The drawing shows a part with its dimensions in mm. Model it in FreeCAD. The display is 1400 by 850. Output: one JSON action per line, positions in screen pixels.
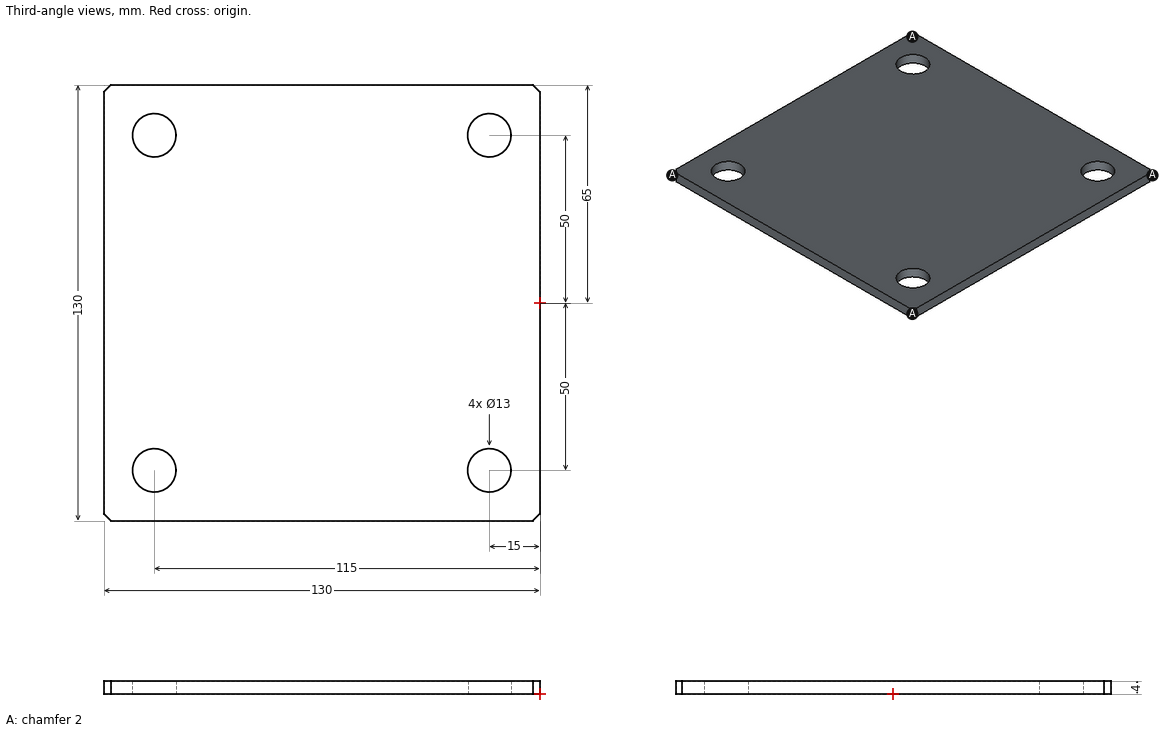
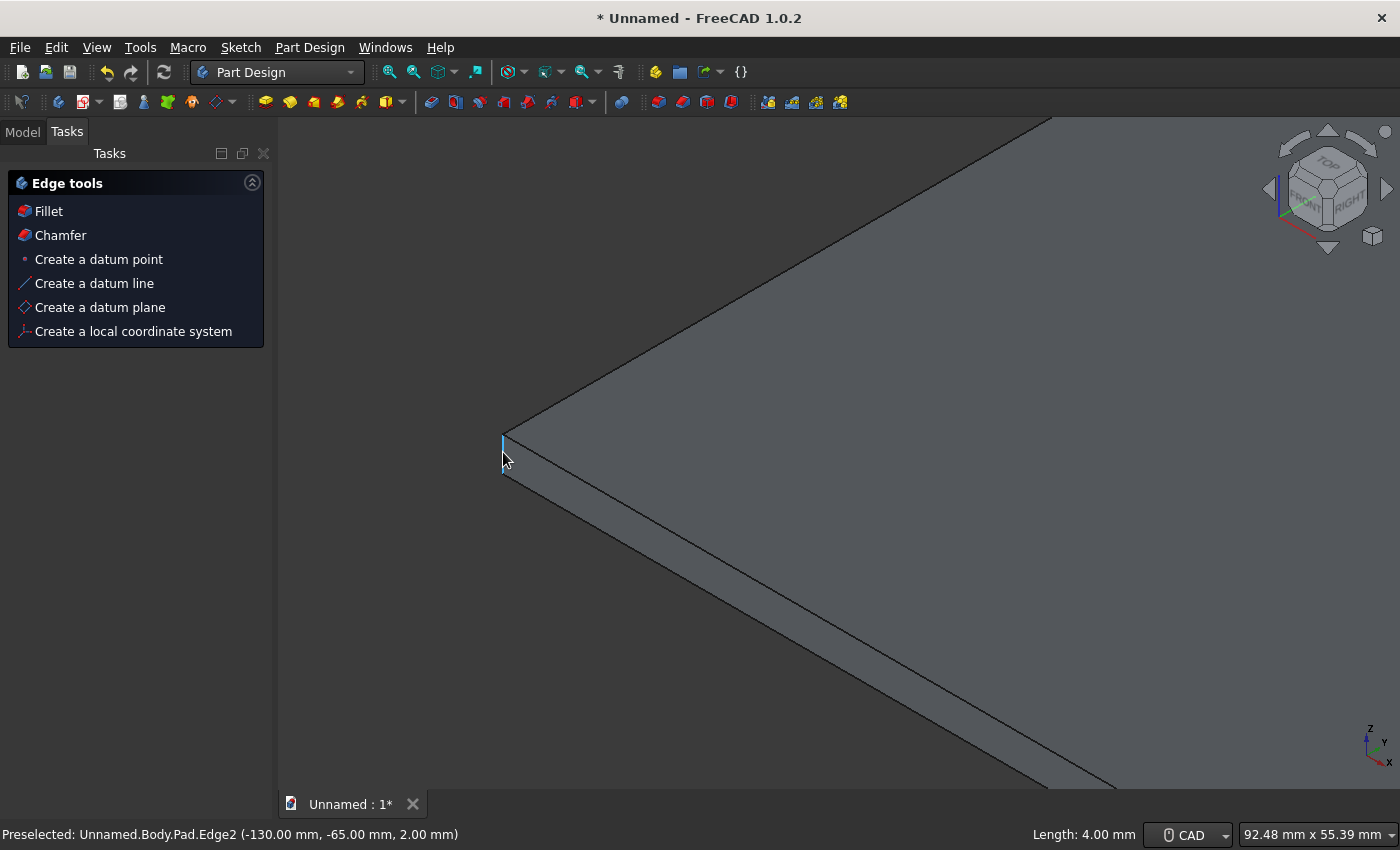
{"action": "left_click", "coordinate": [390, 72]}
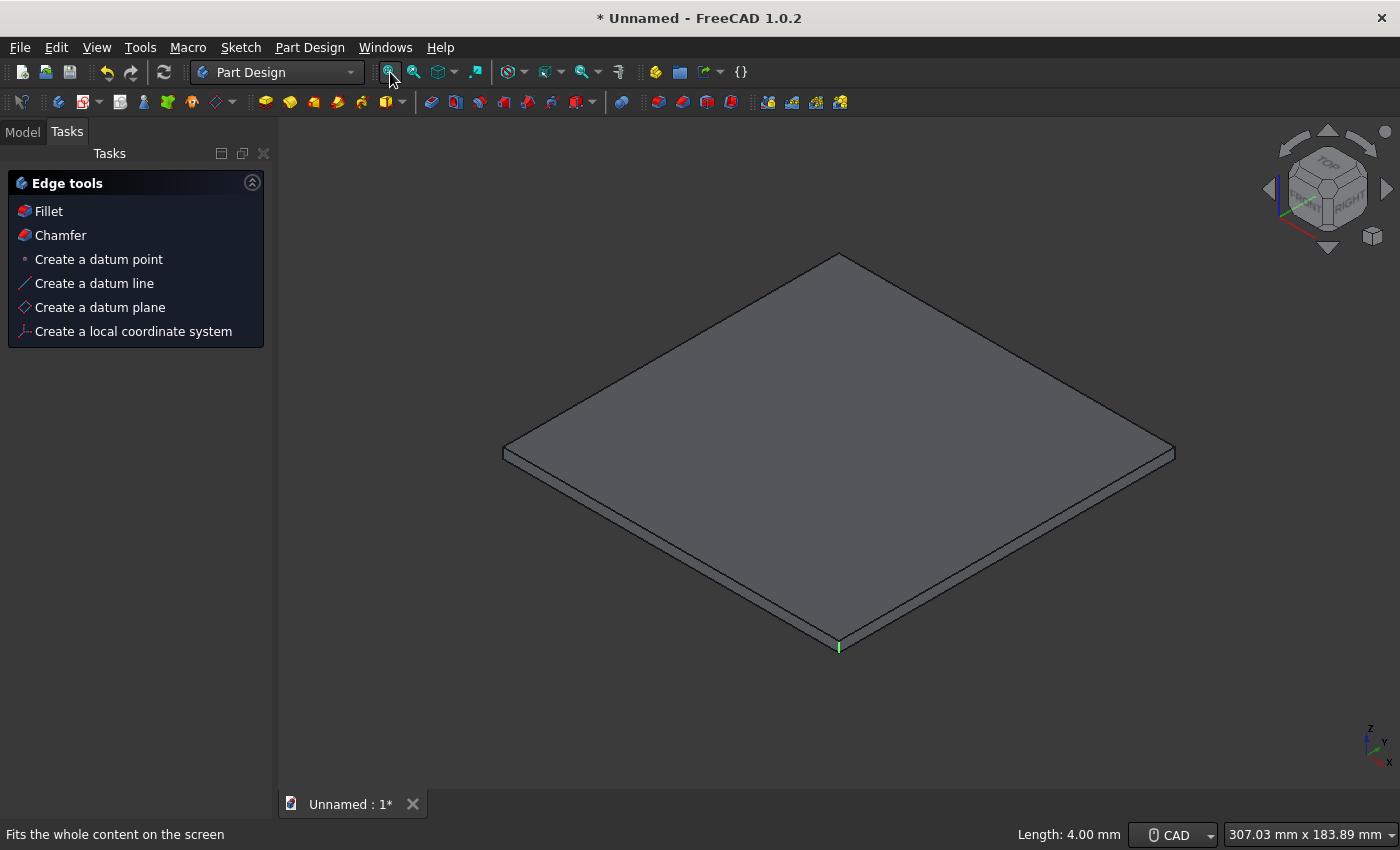
{"action": "key", "text": "2"}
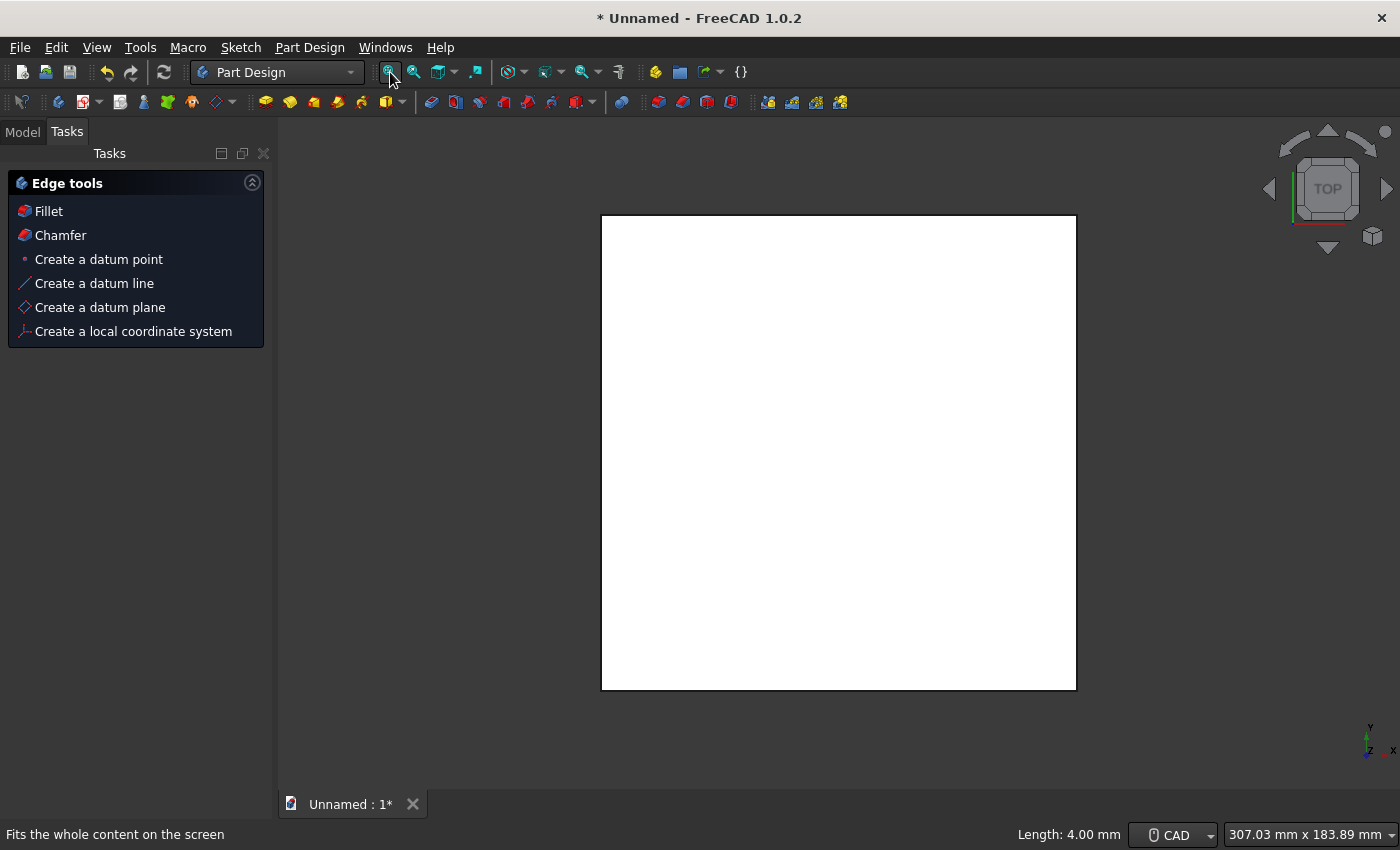
{"action": "scroll", "coordinate": [601, 690], "scroll_direction": "up", "scroll_amount": 6}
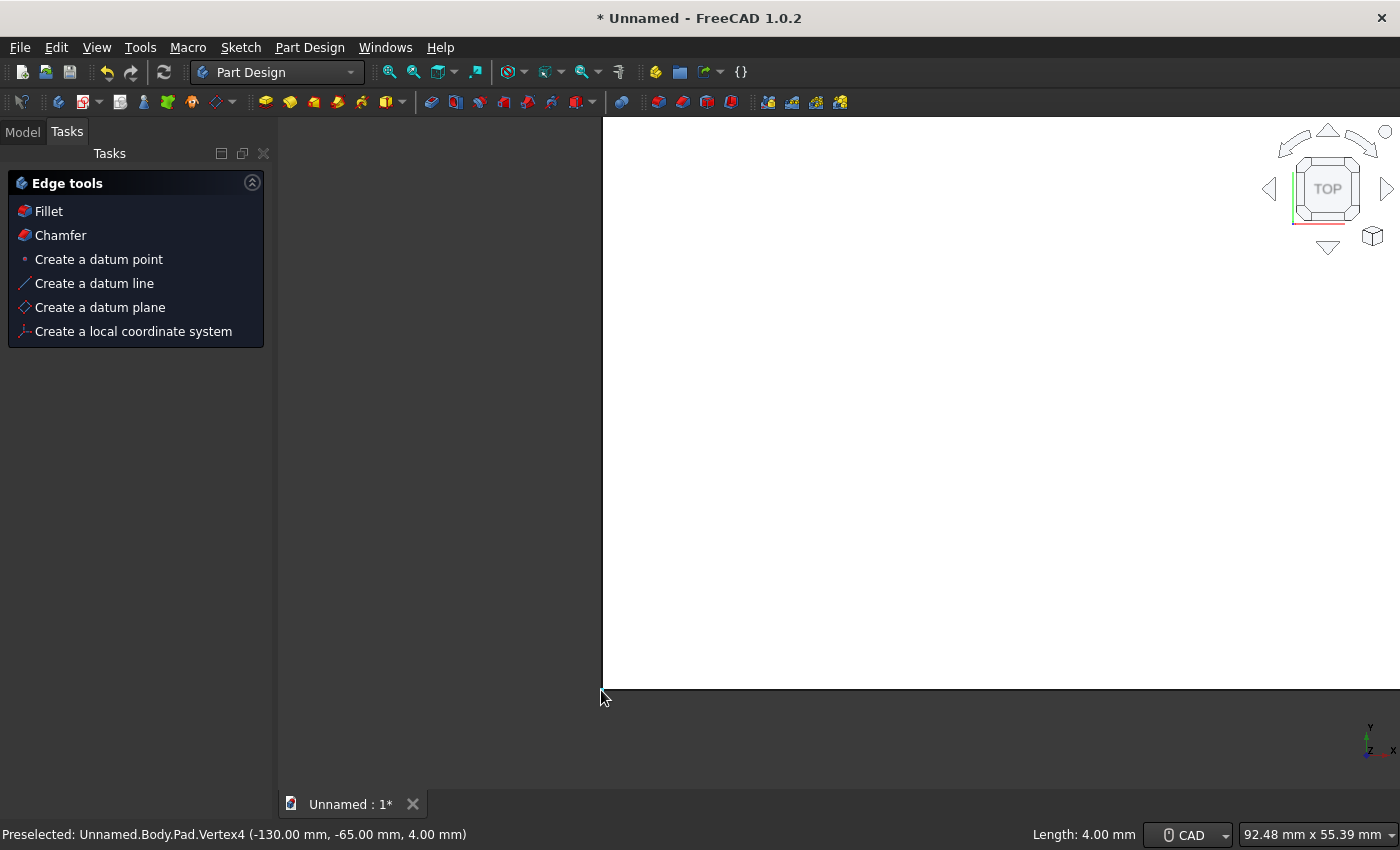
{"action": "left_click", "coordinate": [390, 72]}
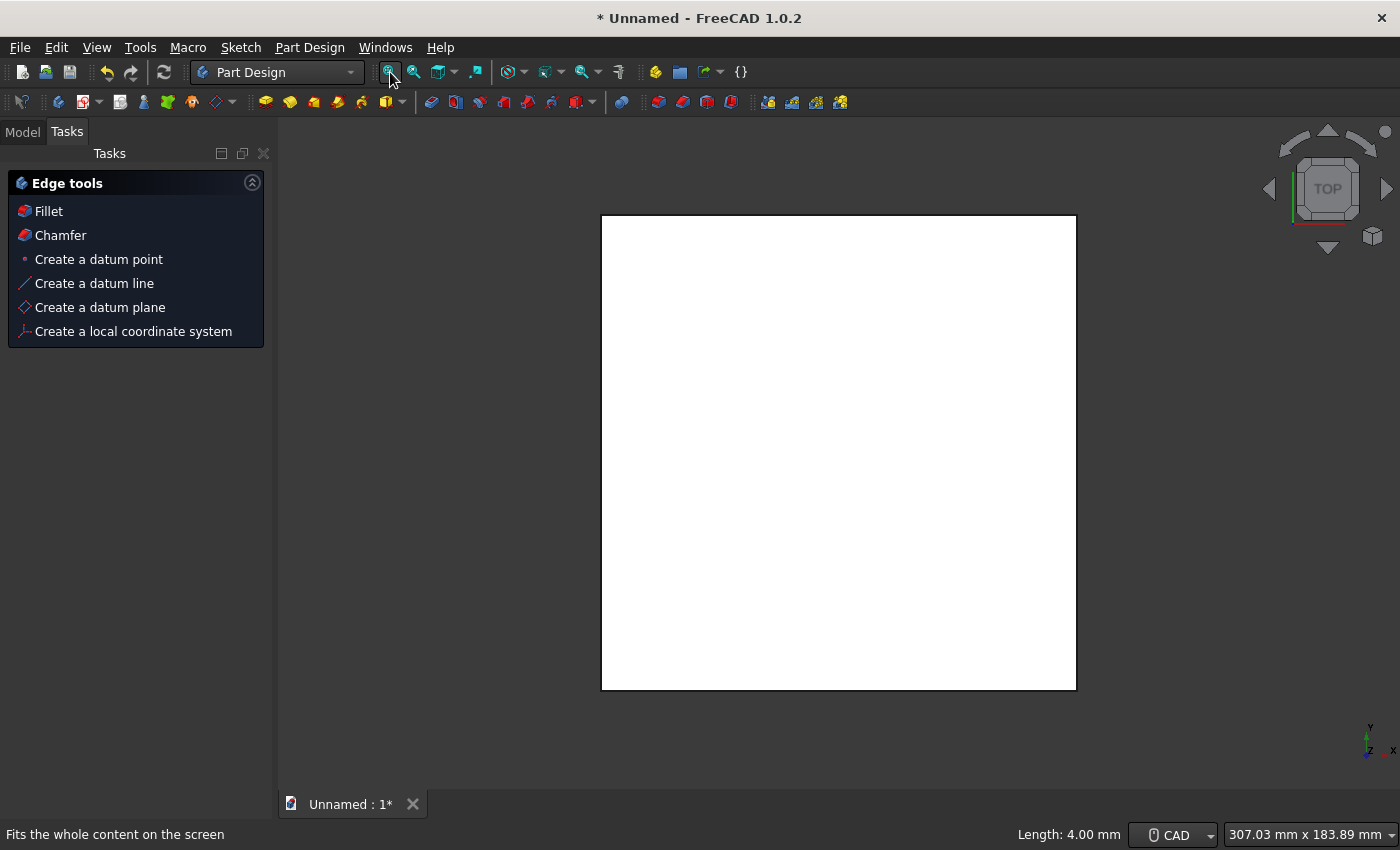
{"action": "key", "text": "1"}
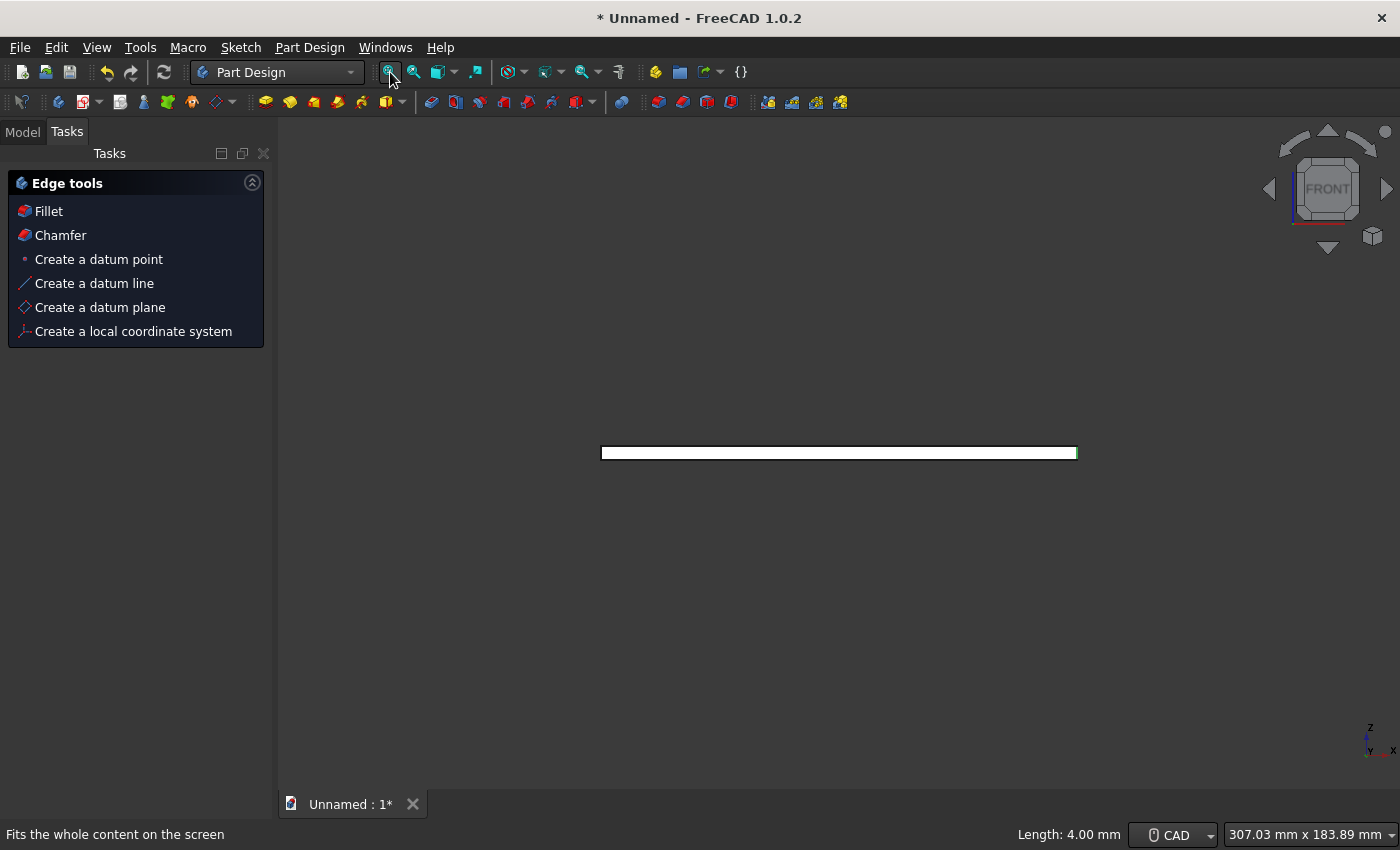
{"action": "left_click", "coordinate": [390, 72]}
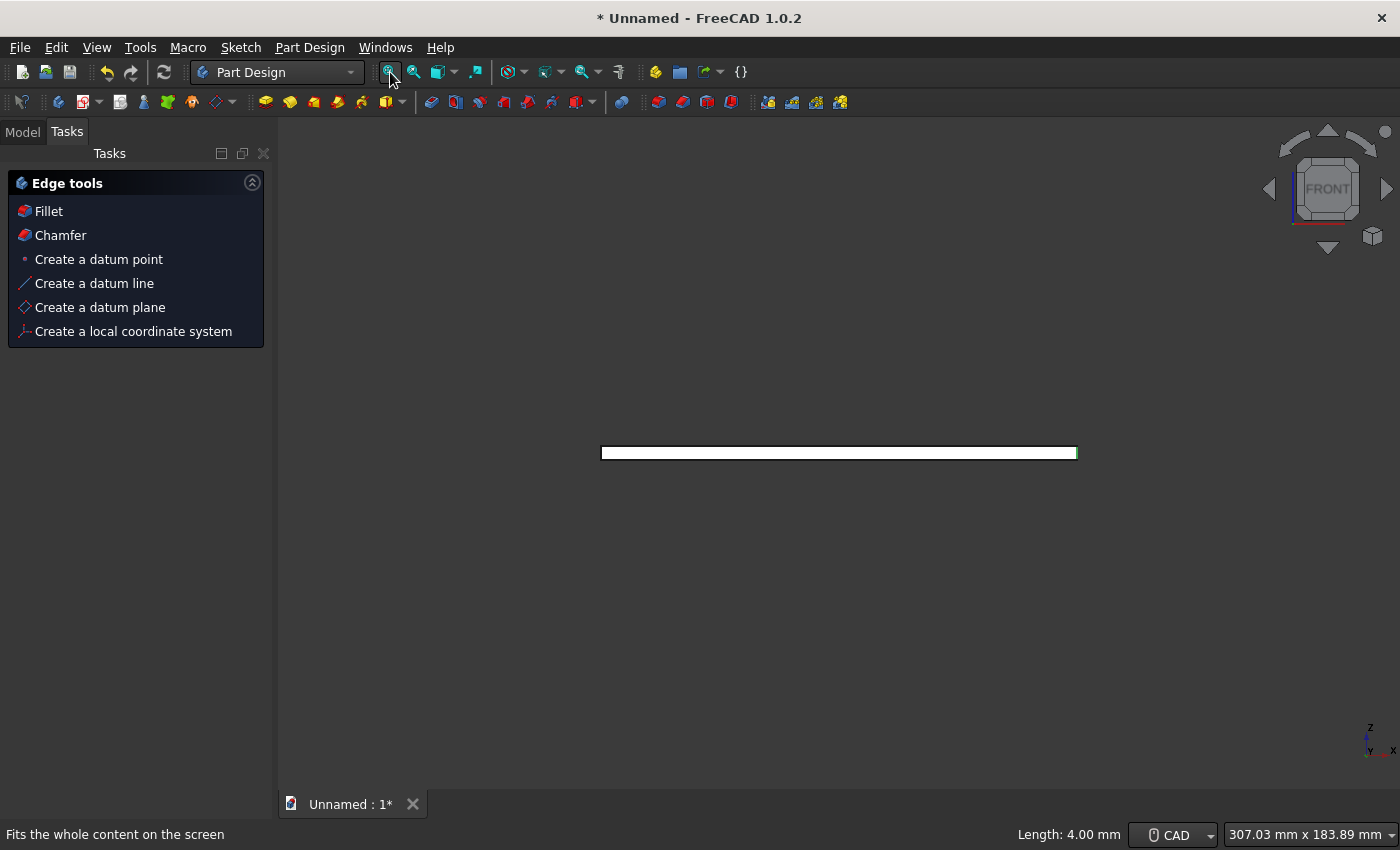
{"action": "left_click", "coordinate": [601, 452], "text": "ctrl"}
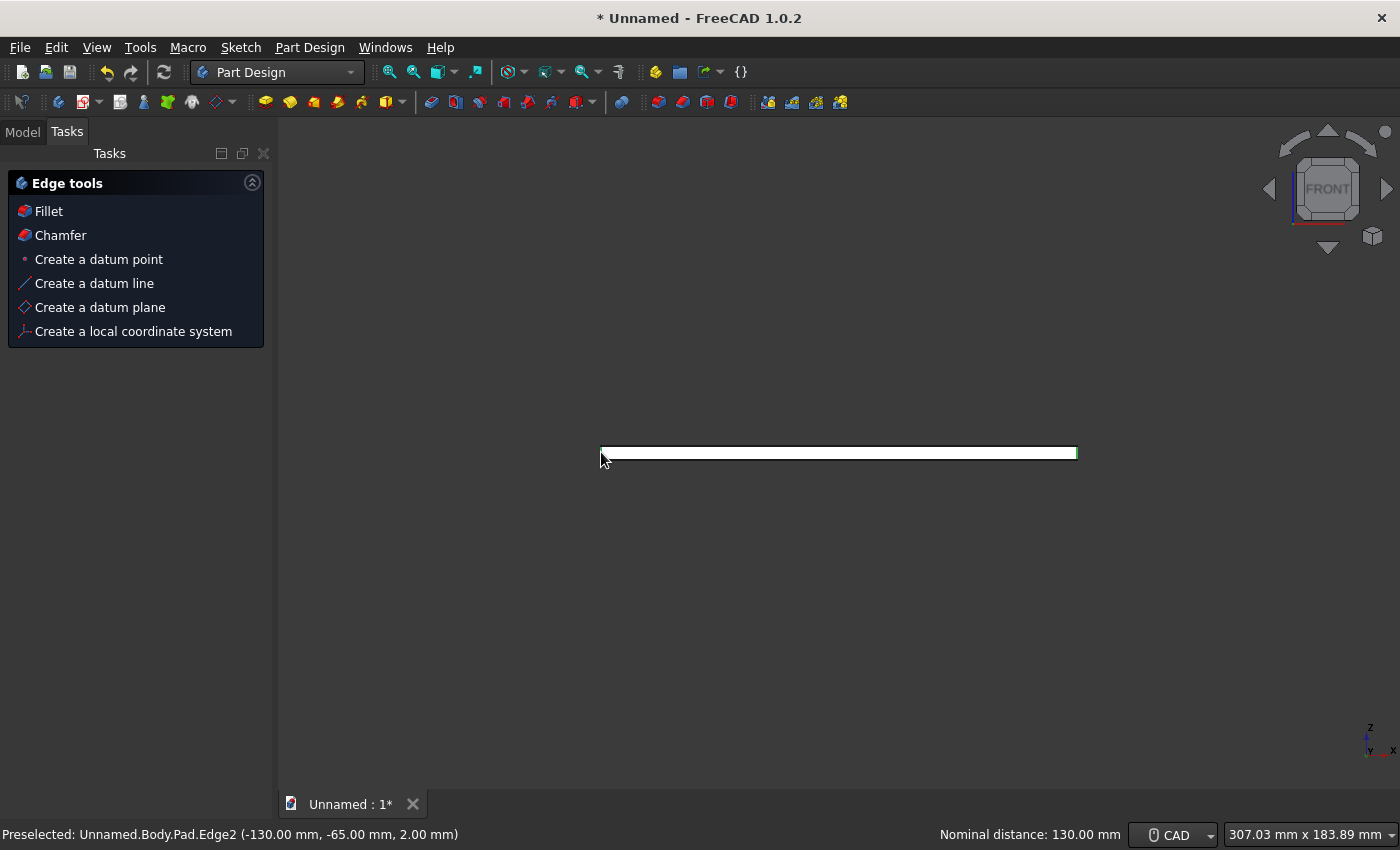
{"action": "scroll", "coordinate": [601, 452], "scroll_direction": "up", "scroll_amount": 6}